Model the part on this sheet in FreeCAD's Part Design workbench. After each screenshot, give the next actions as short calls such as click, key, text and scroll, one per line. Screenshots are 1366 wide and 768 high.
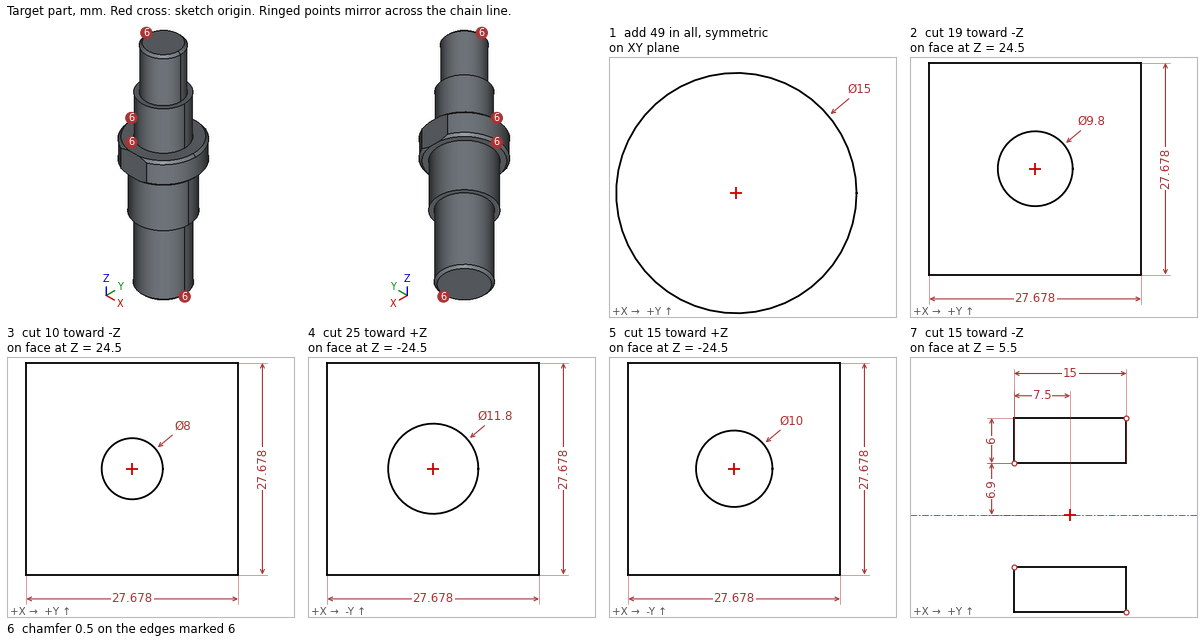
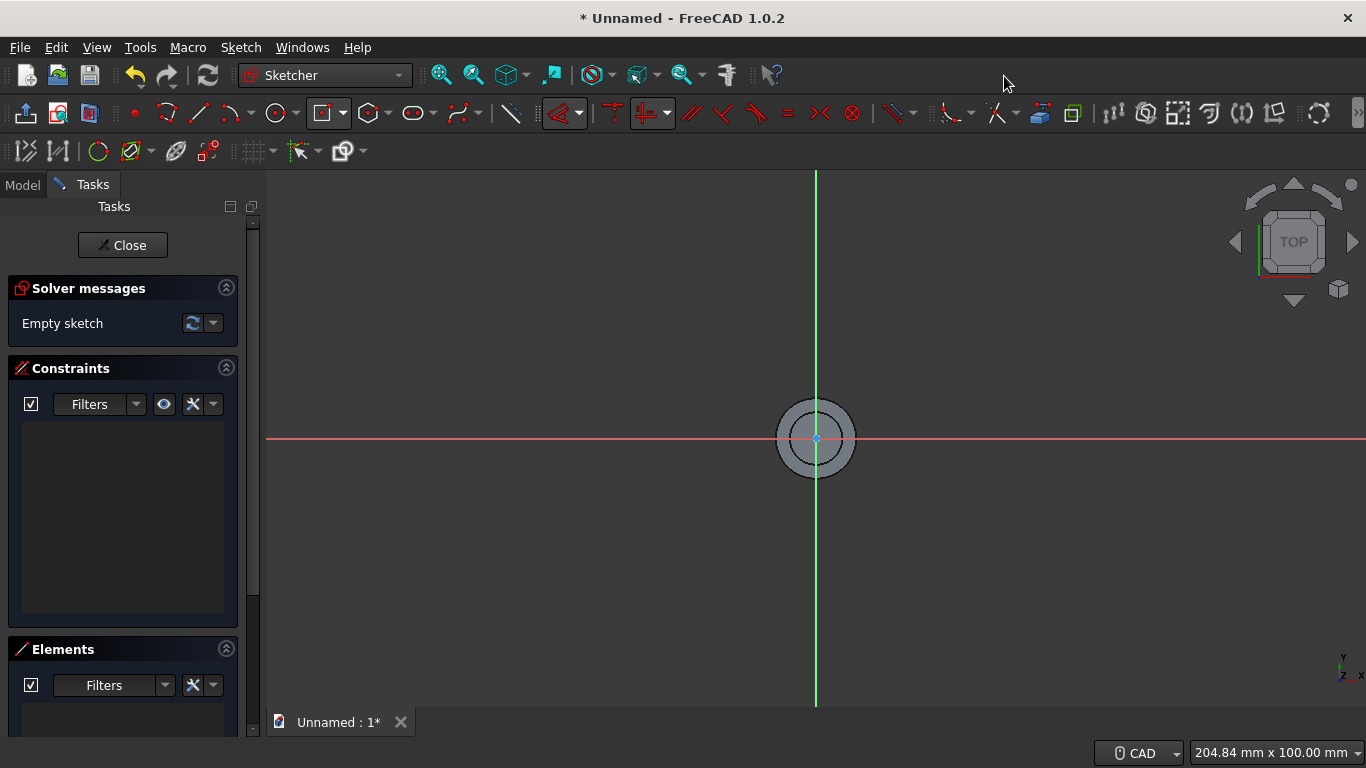
scroll(872, 438, up, 4)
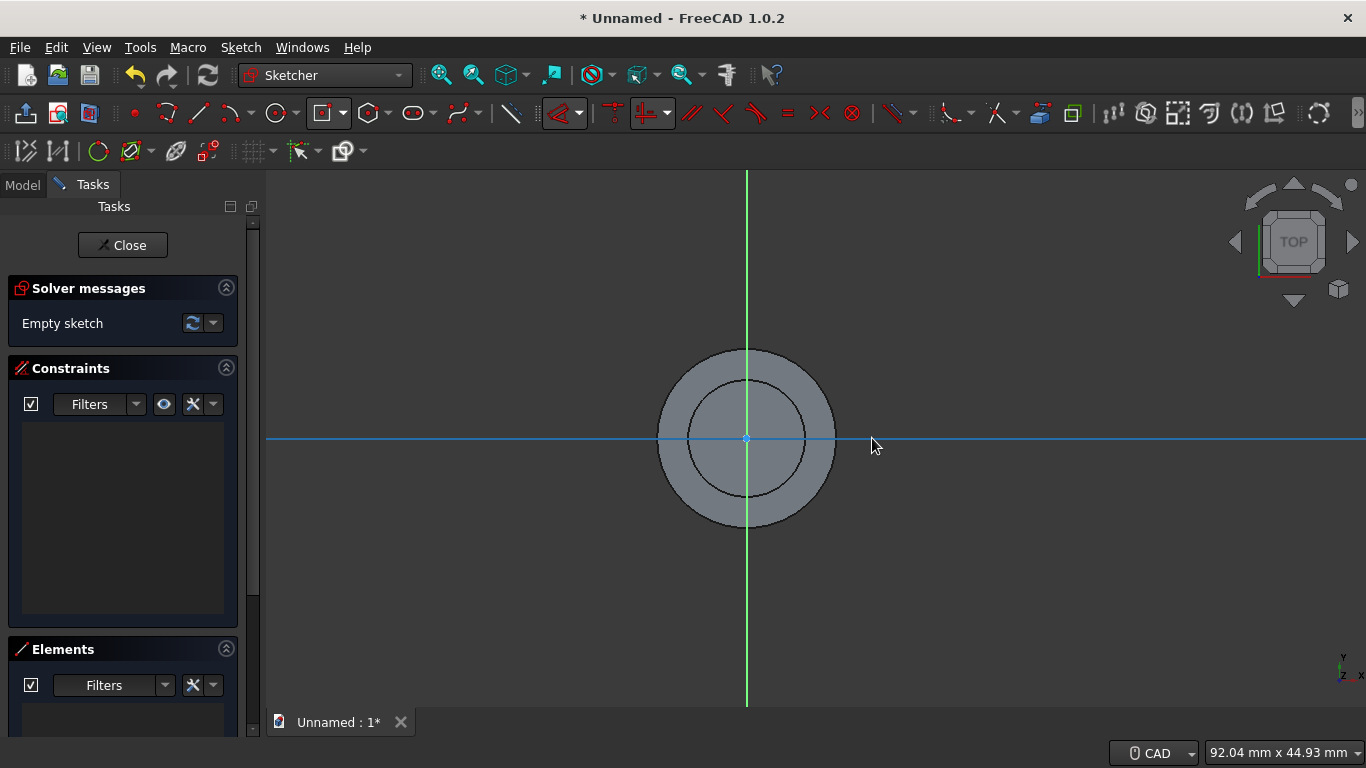
click(322, 114)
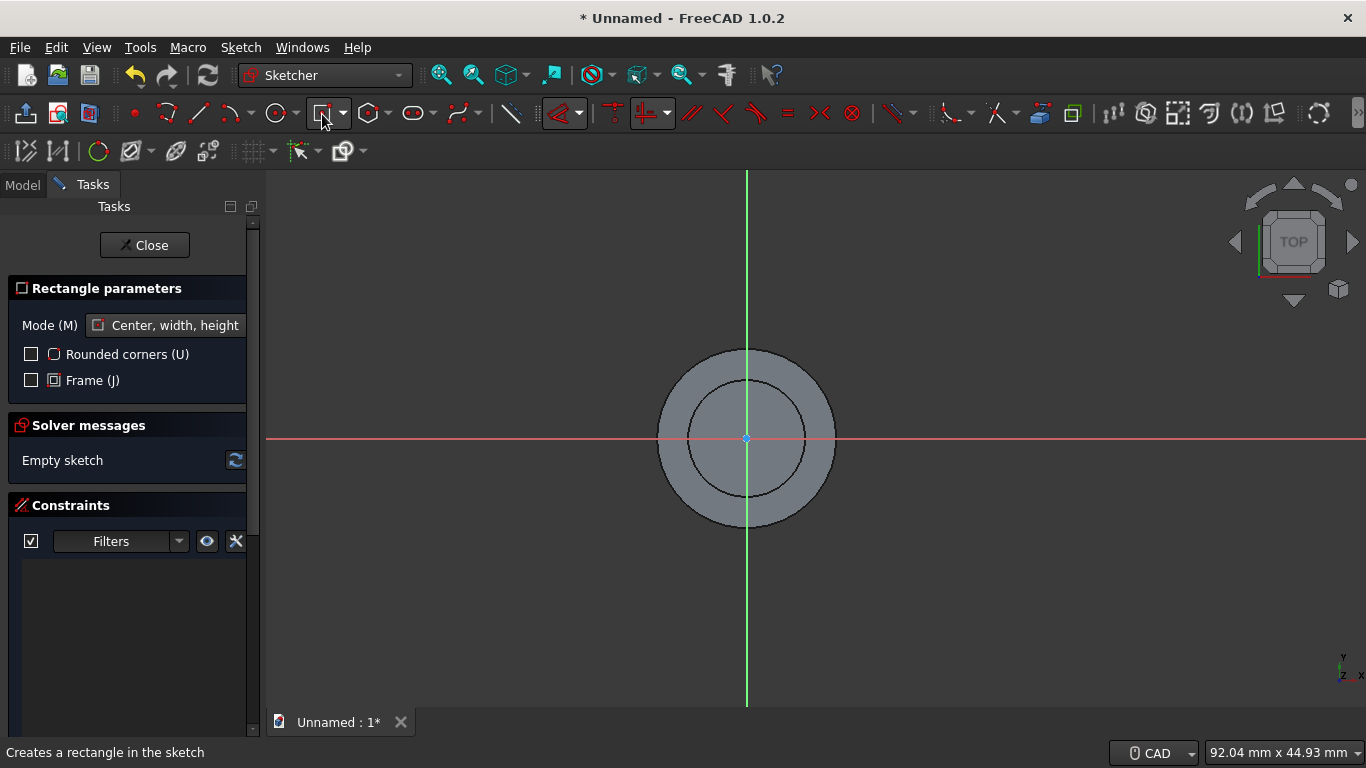
click(747, 438)
click(912, 273)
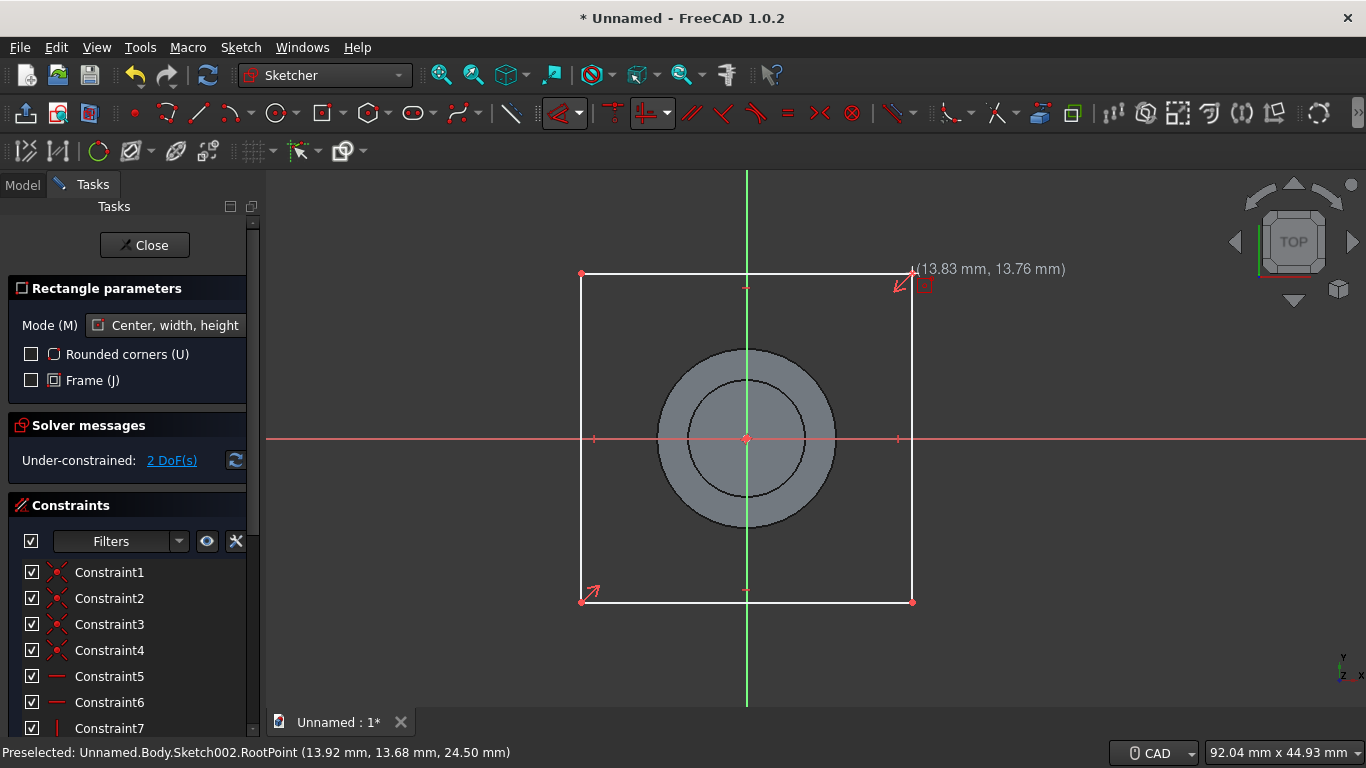
click(276, 114)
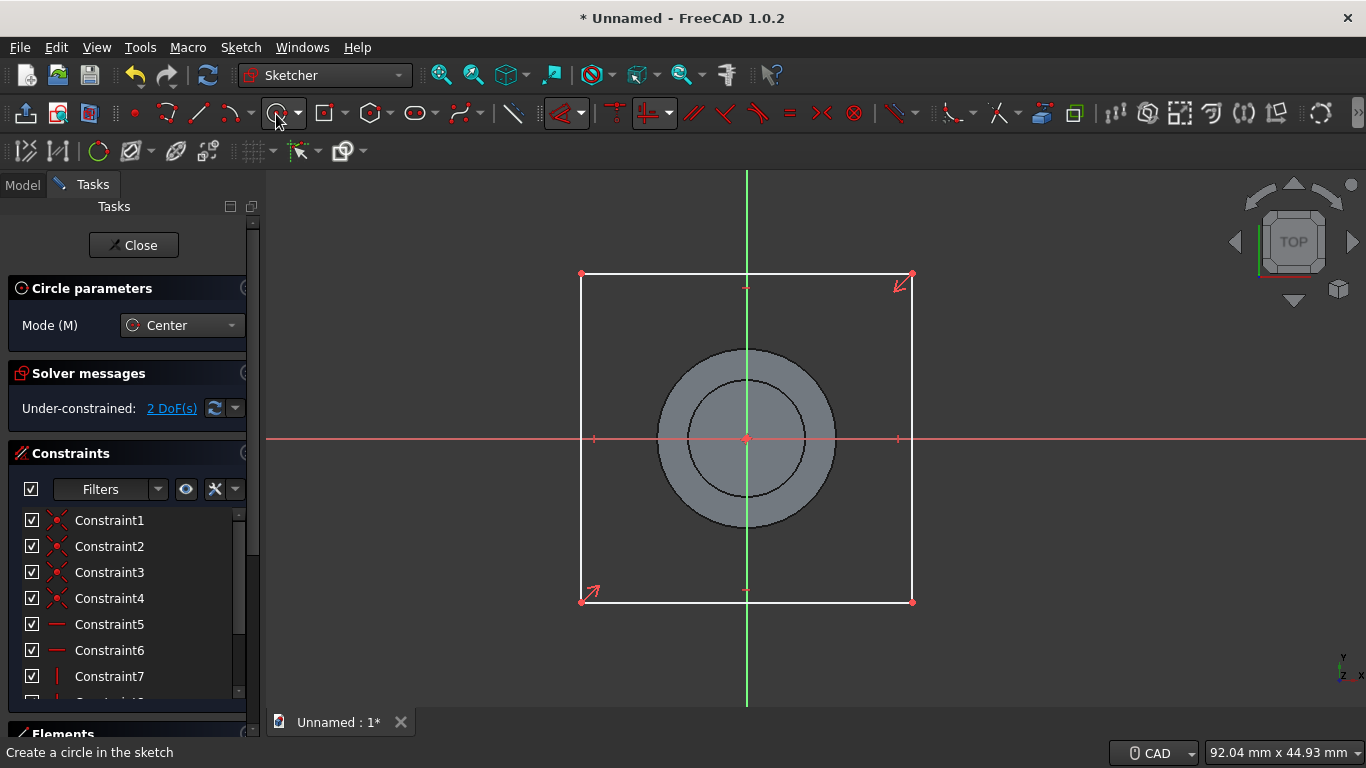
click(747, 438)
click(780, 405)
key(Escape)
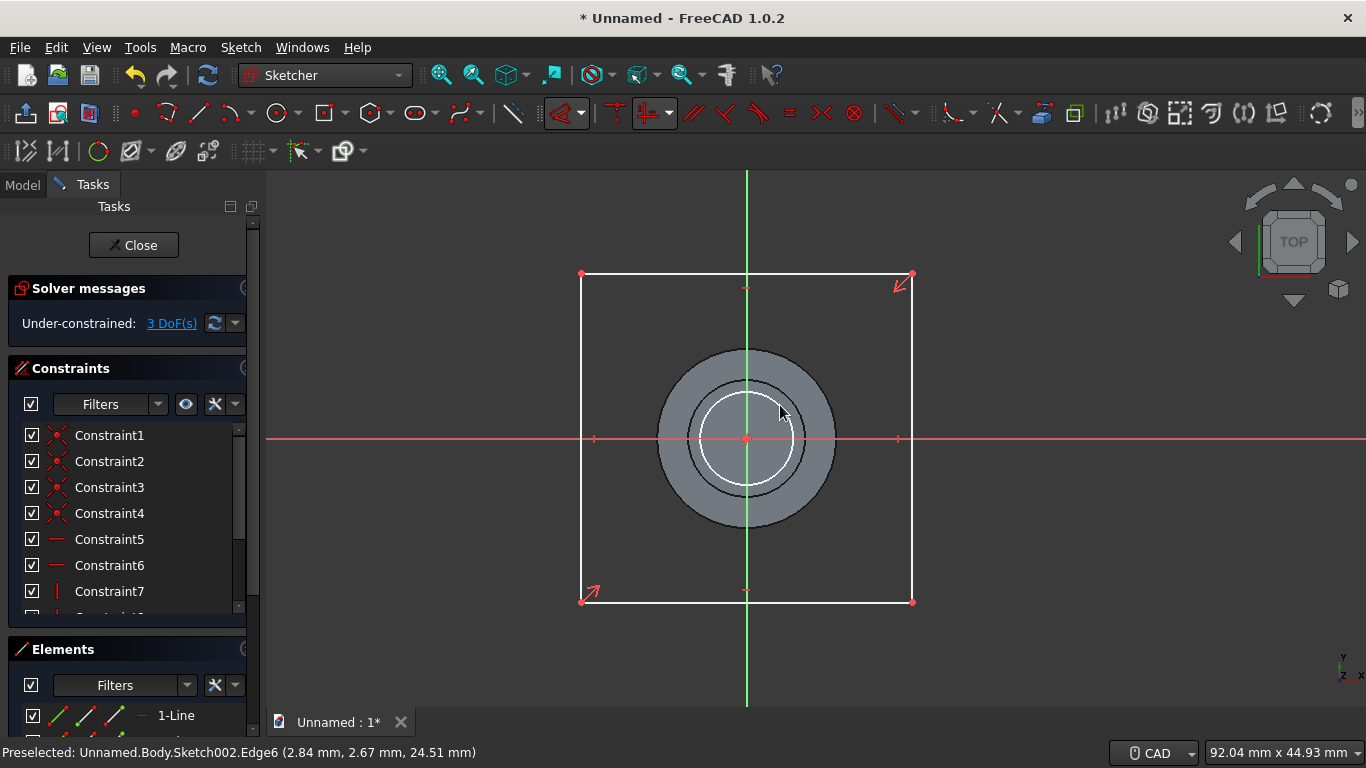
click(779, 405)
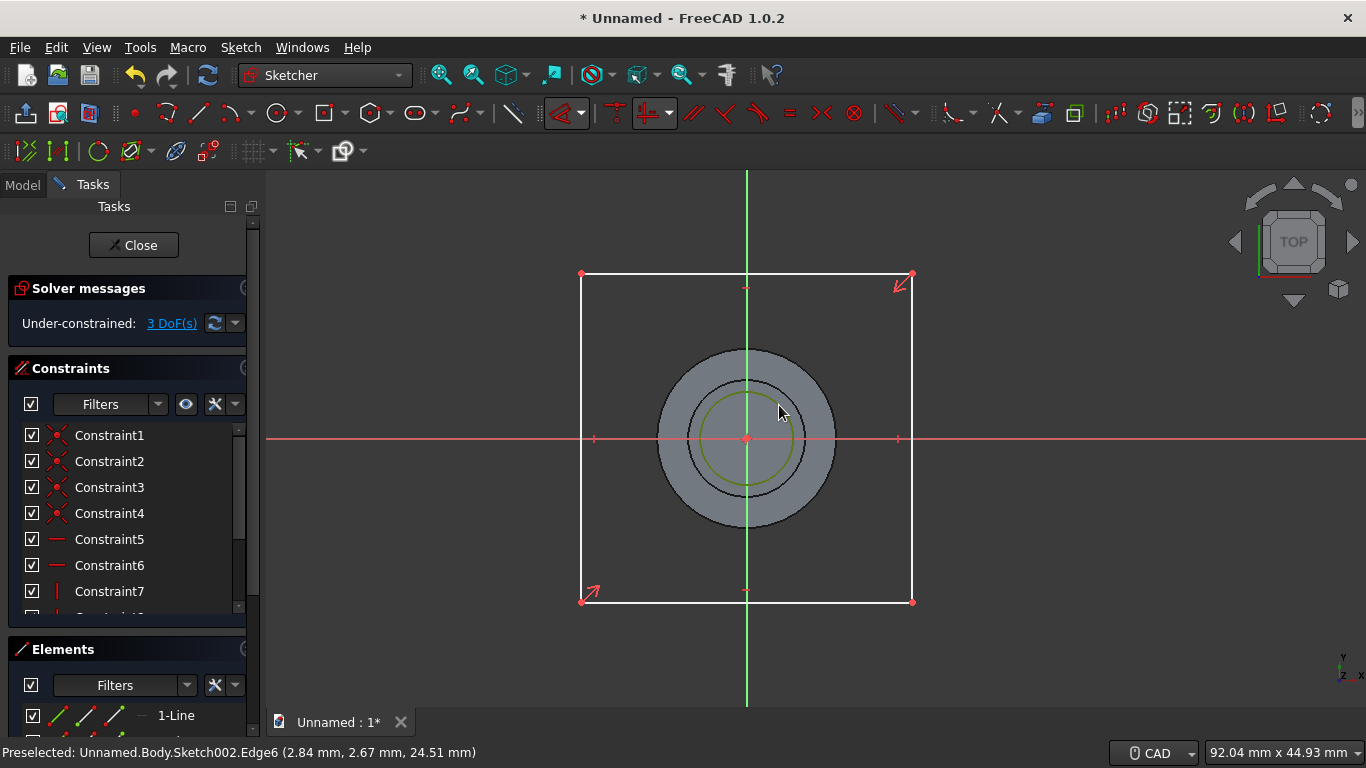
key(k)
key(o)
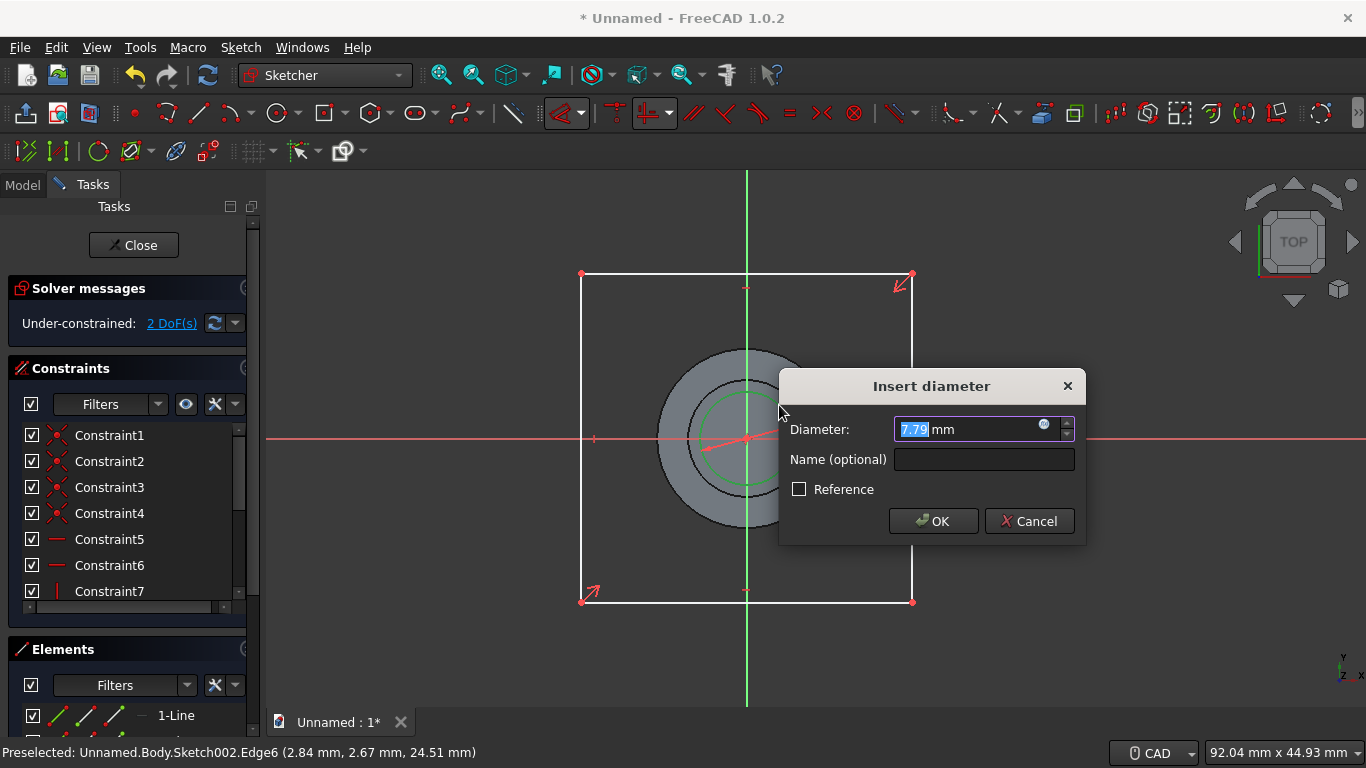
text(8)
key(Return)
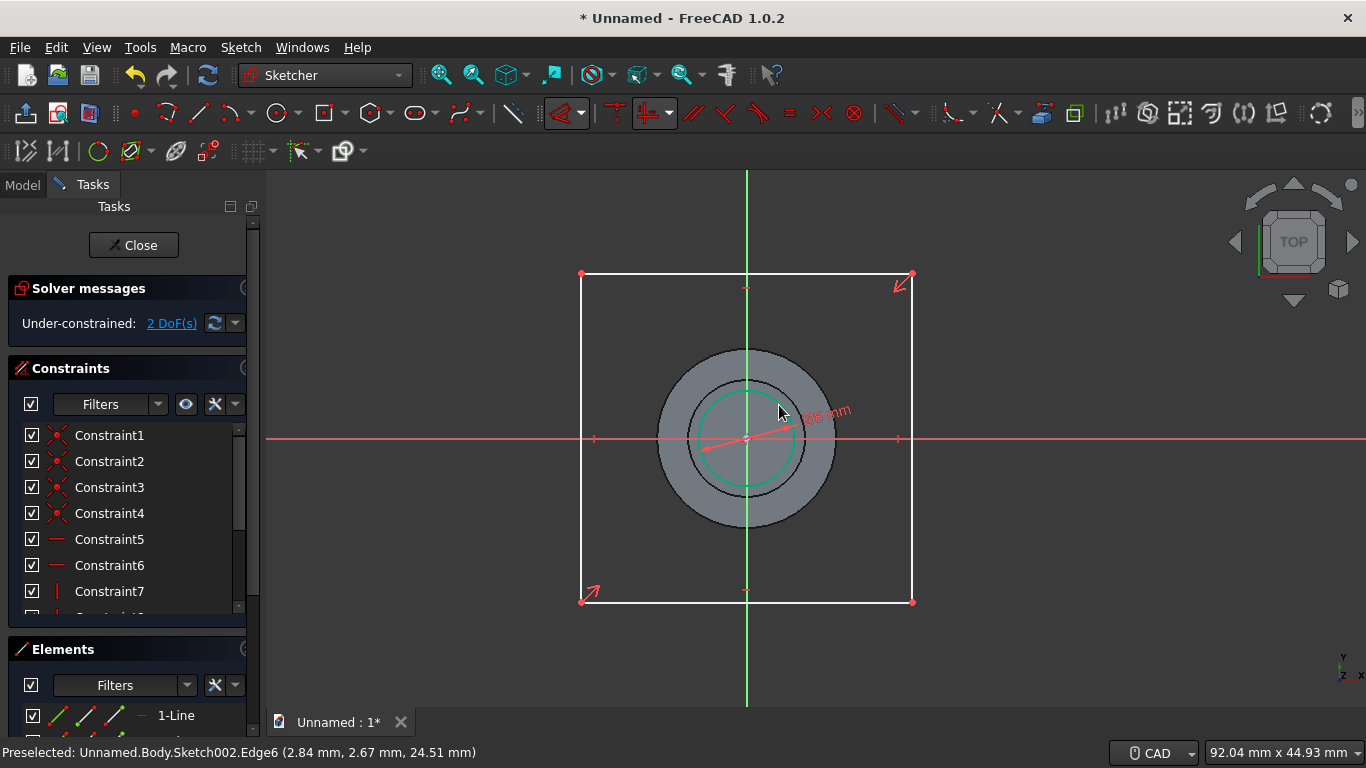
click(681, 603)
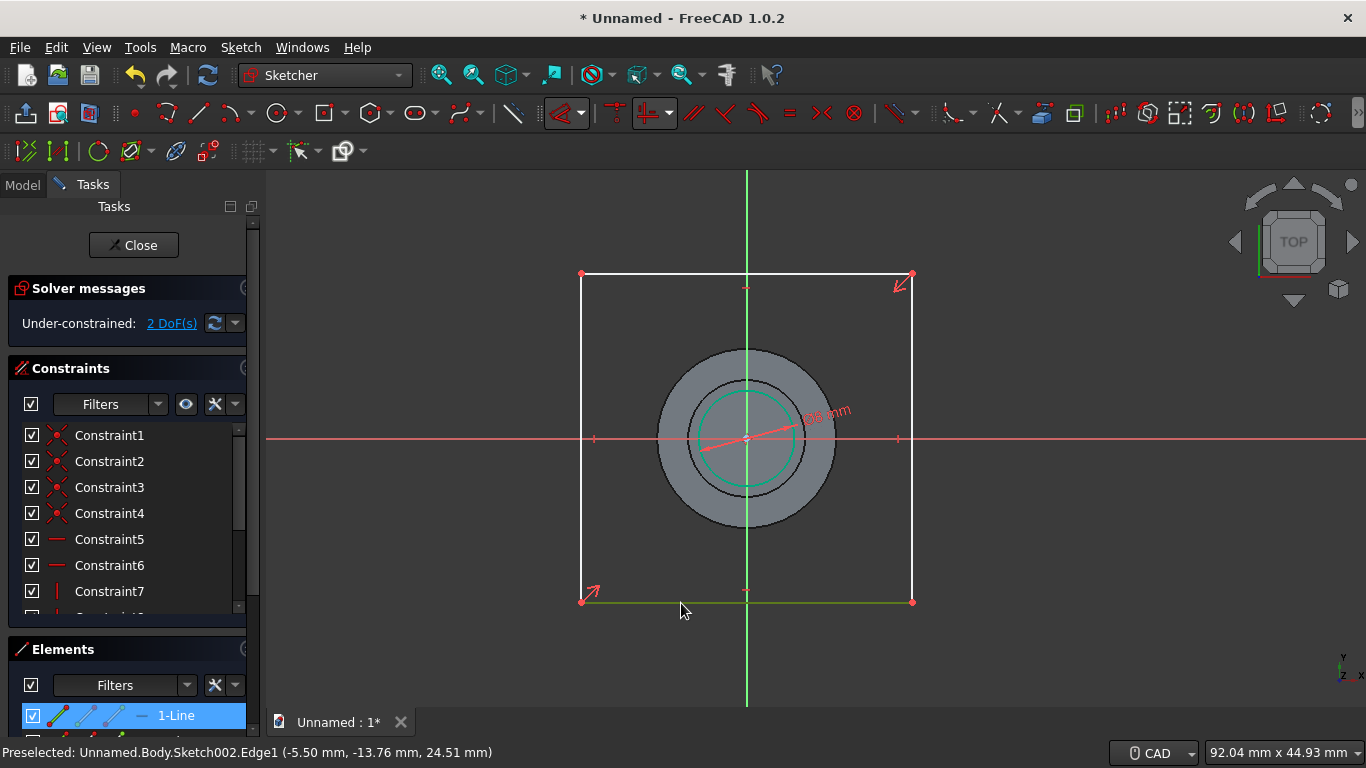
key(l)